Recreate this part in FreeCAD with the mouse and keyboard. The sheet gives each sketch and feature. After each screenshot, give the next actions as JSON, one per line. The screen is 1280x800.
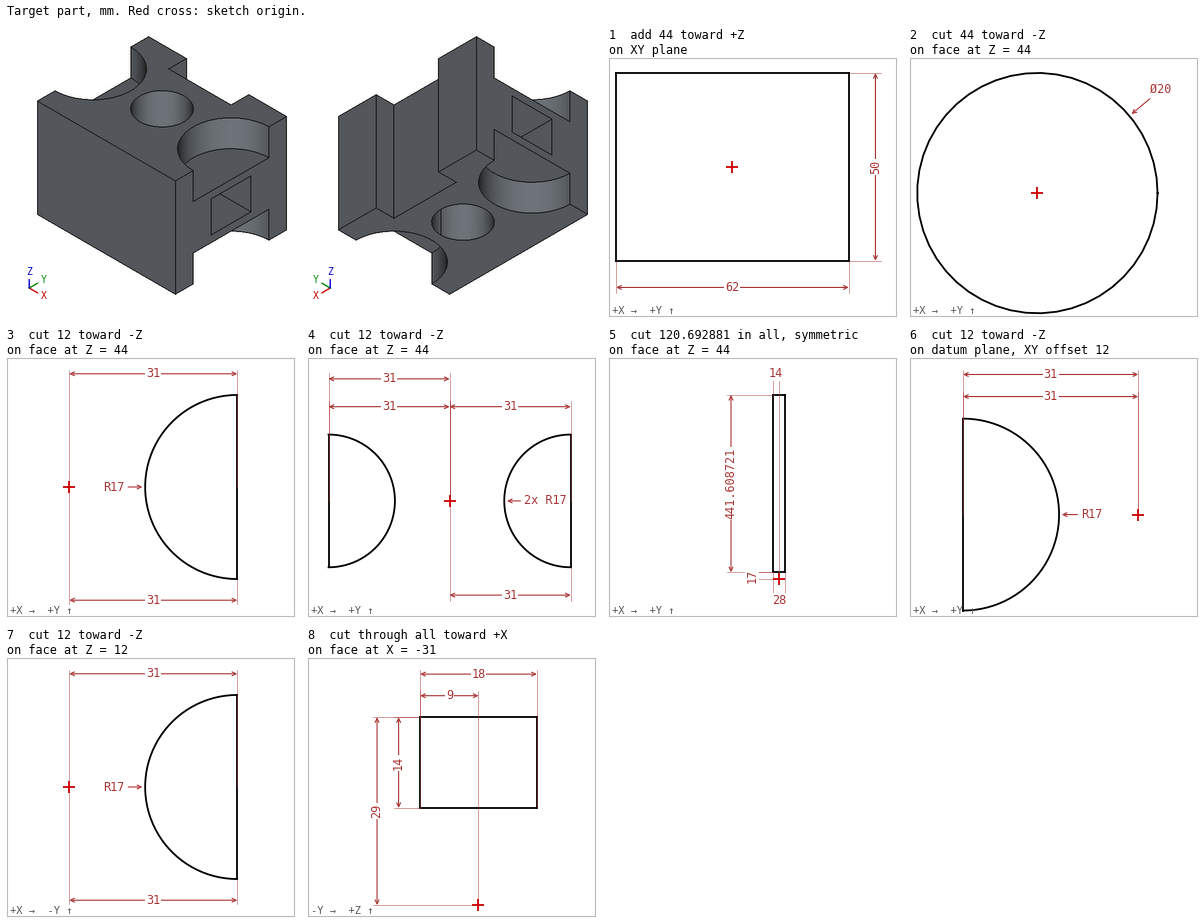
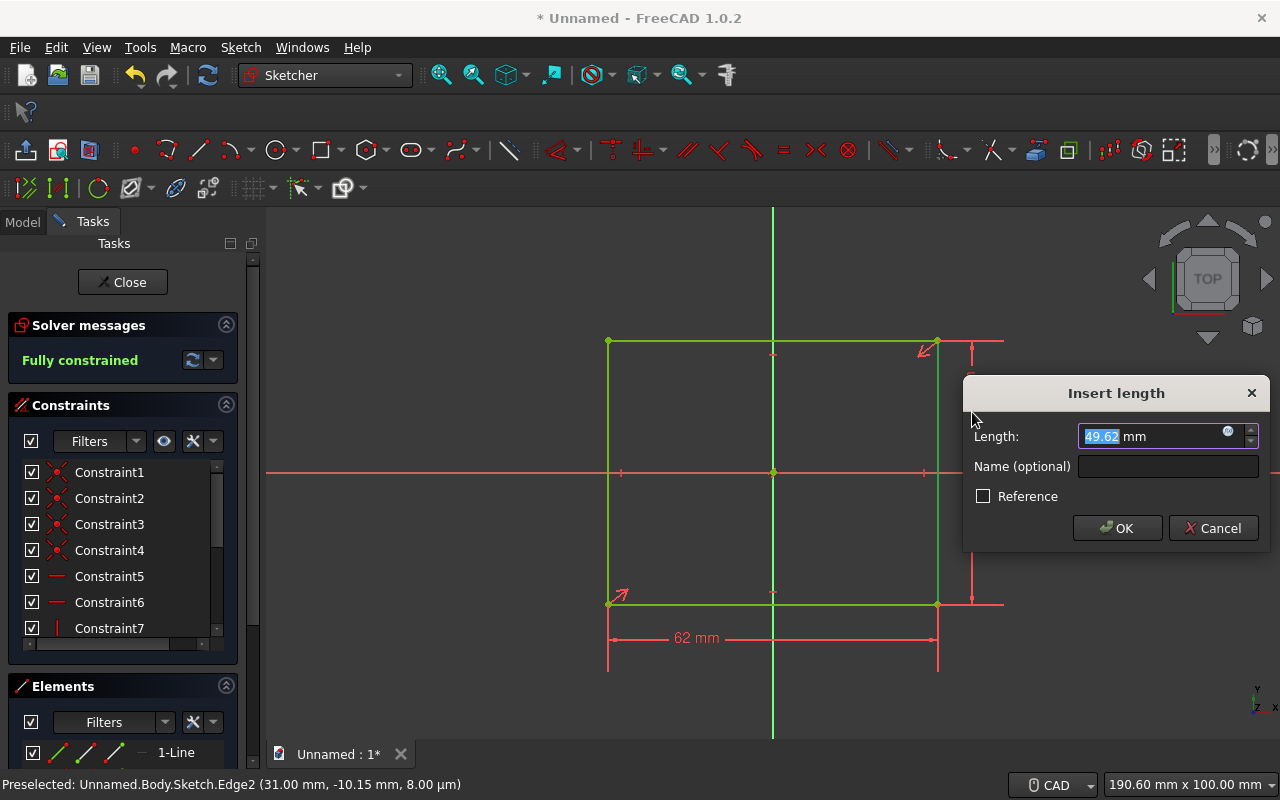
{"action": "type", "text": "50"}
{"action": "key", "text": "Return"}
{"action": "key", "text": "Escape"}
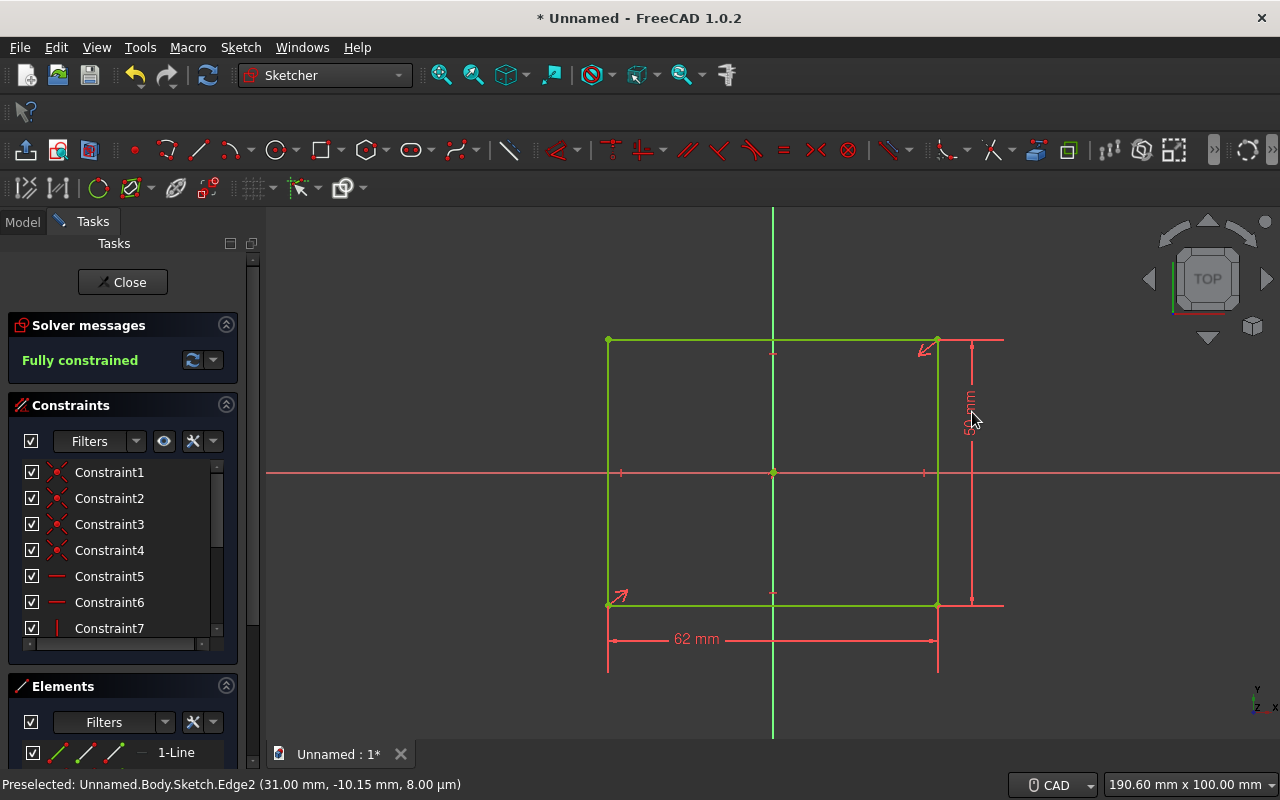
{"action": "left_click", "coordinate": [123, 282]}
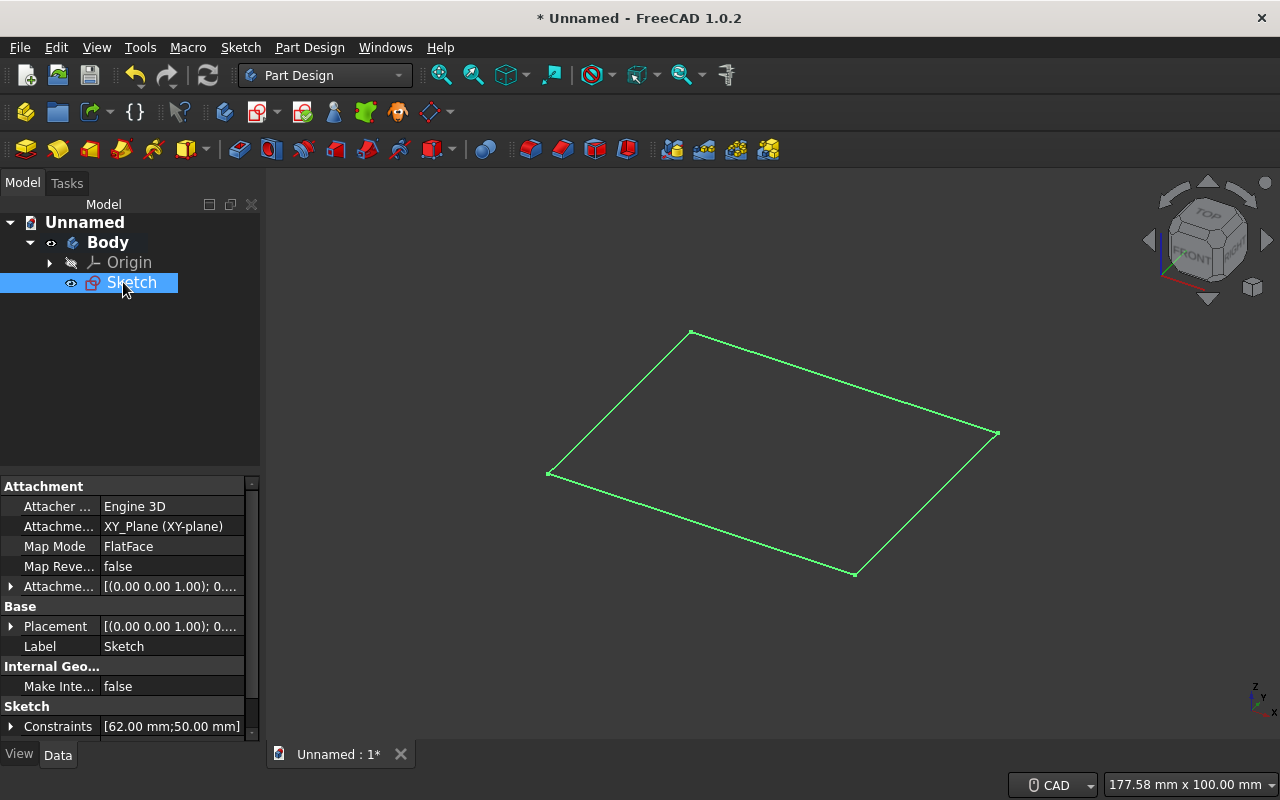
{"action": "left_click", "coordinate": [26, 150]}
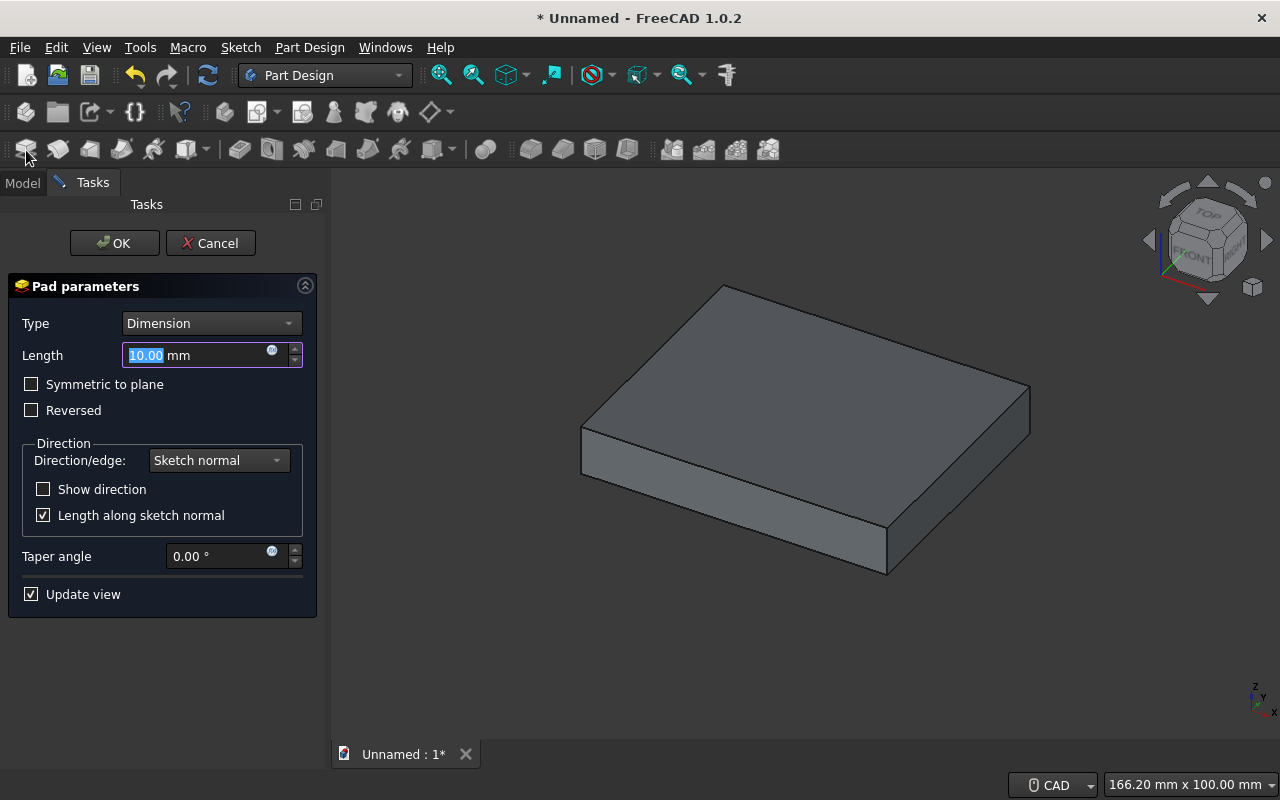
{"action": "type", "text": "44"}
{"action": "key", "text": "Tab"}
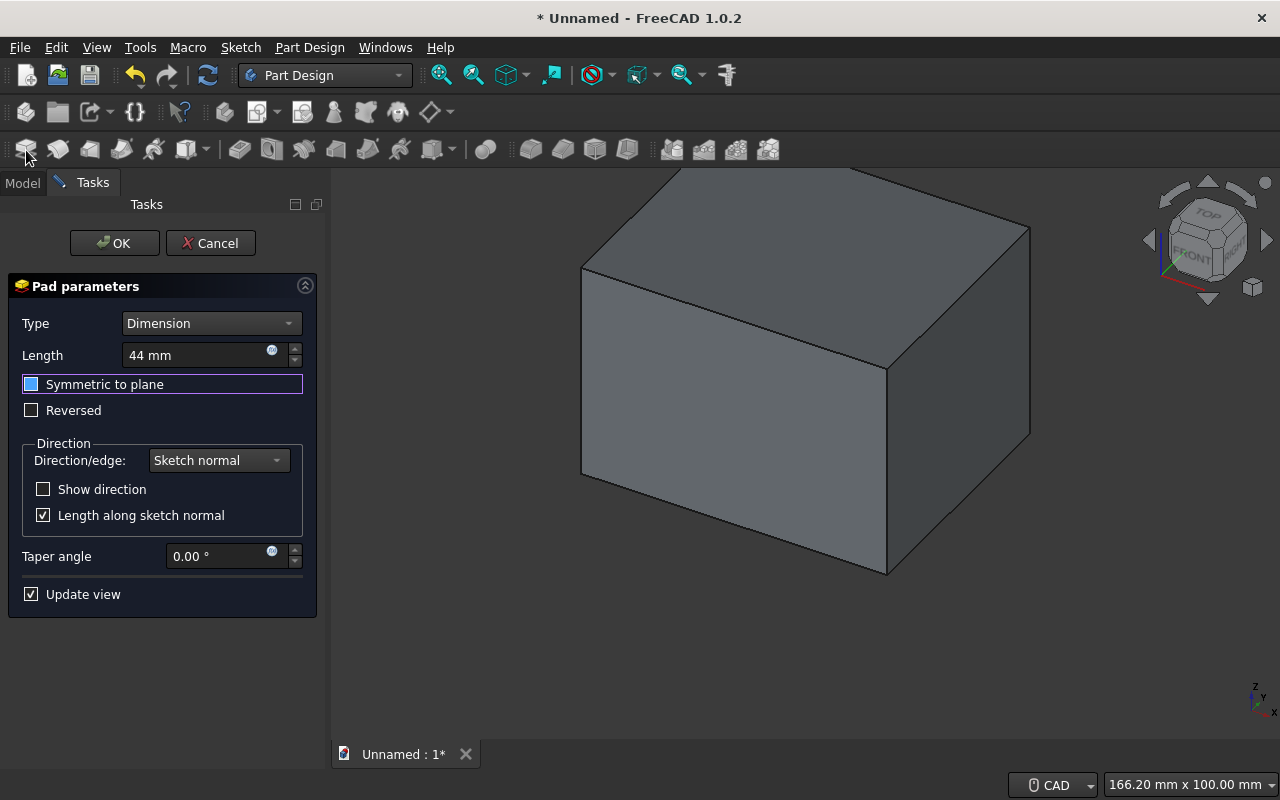
{"action": "left_click", "coordinate": [115, 243]}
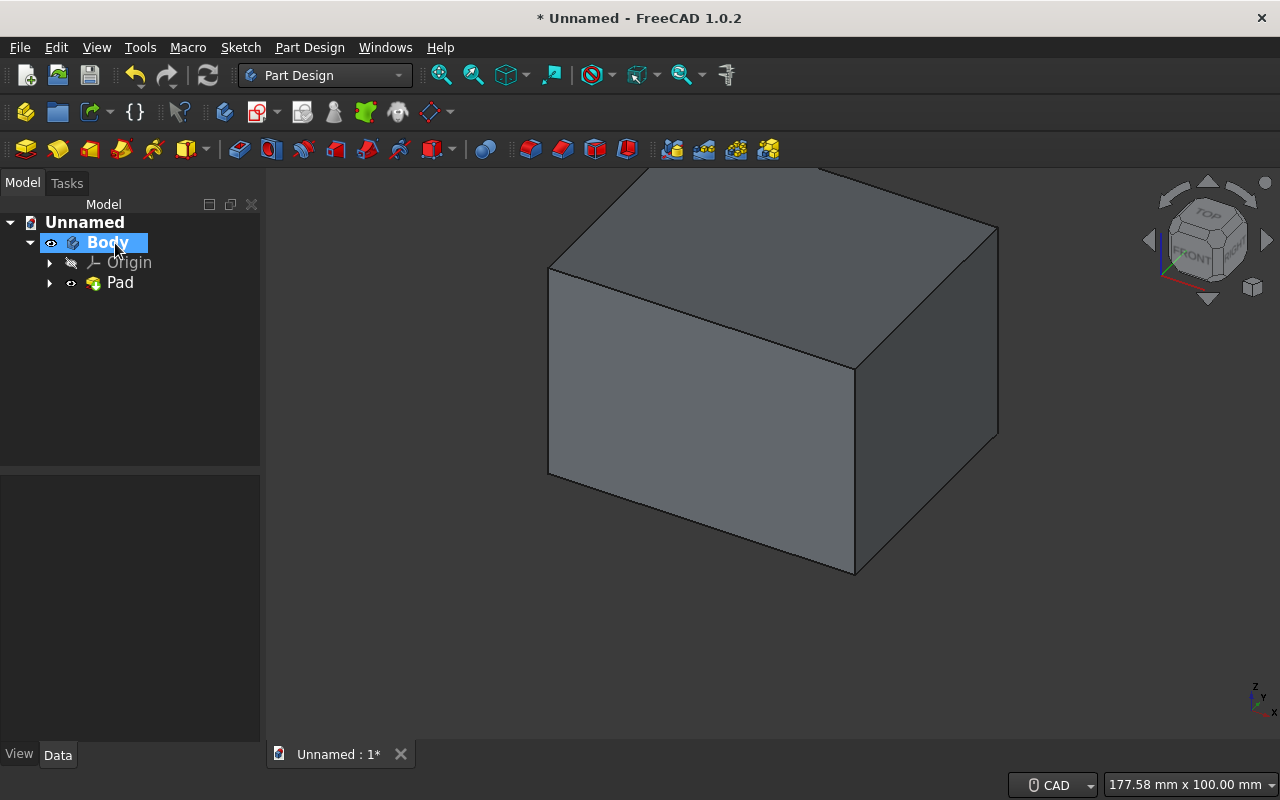
{"action": "key", "text": "v f"}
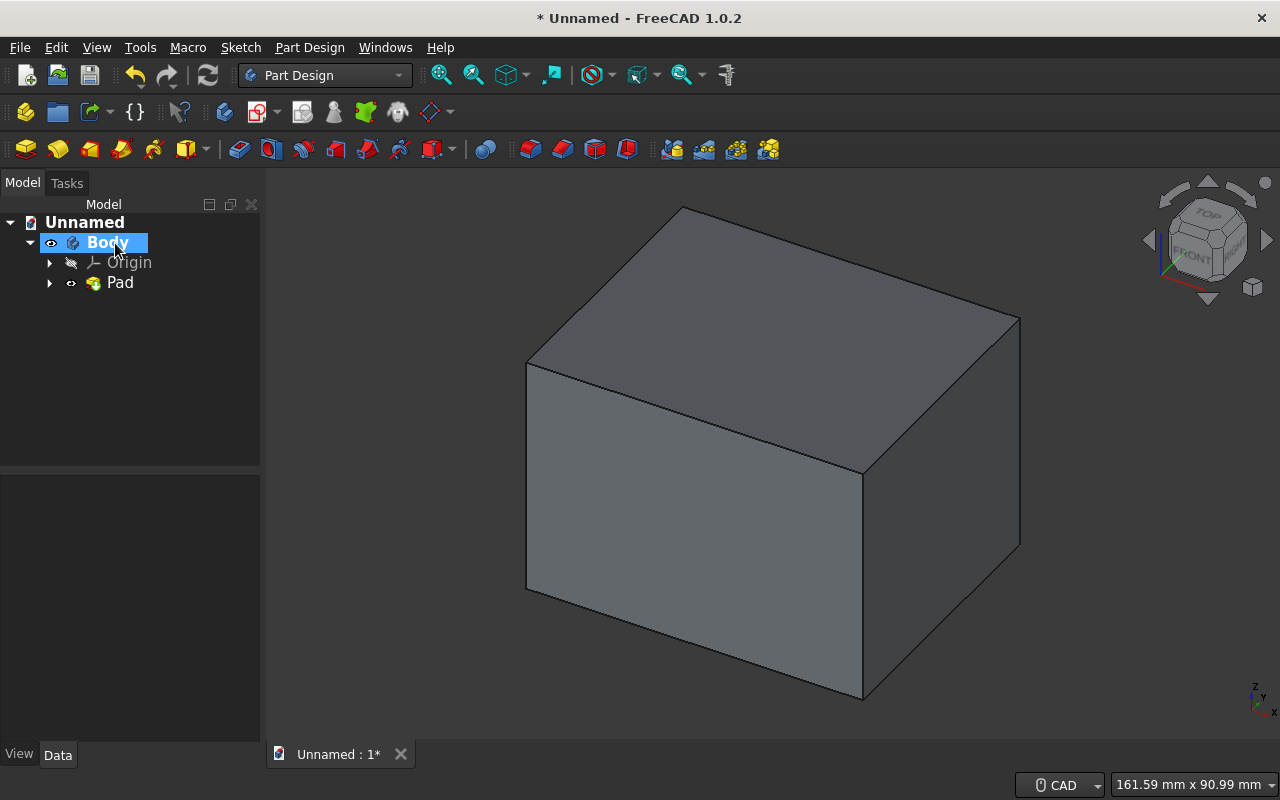
{"action": "left_click", "coordinate": [773, 339]}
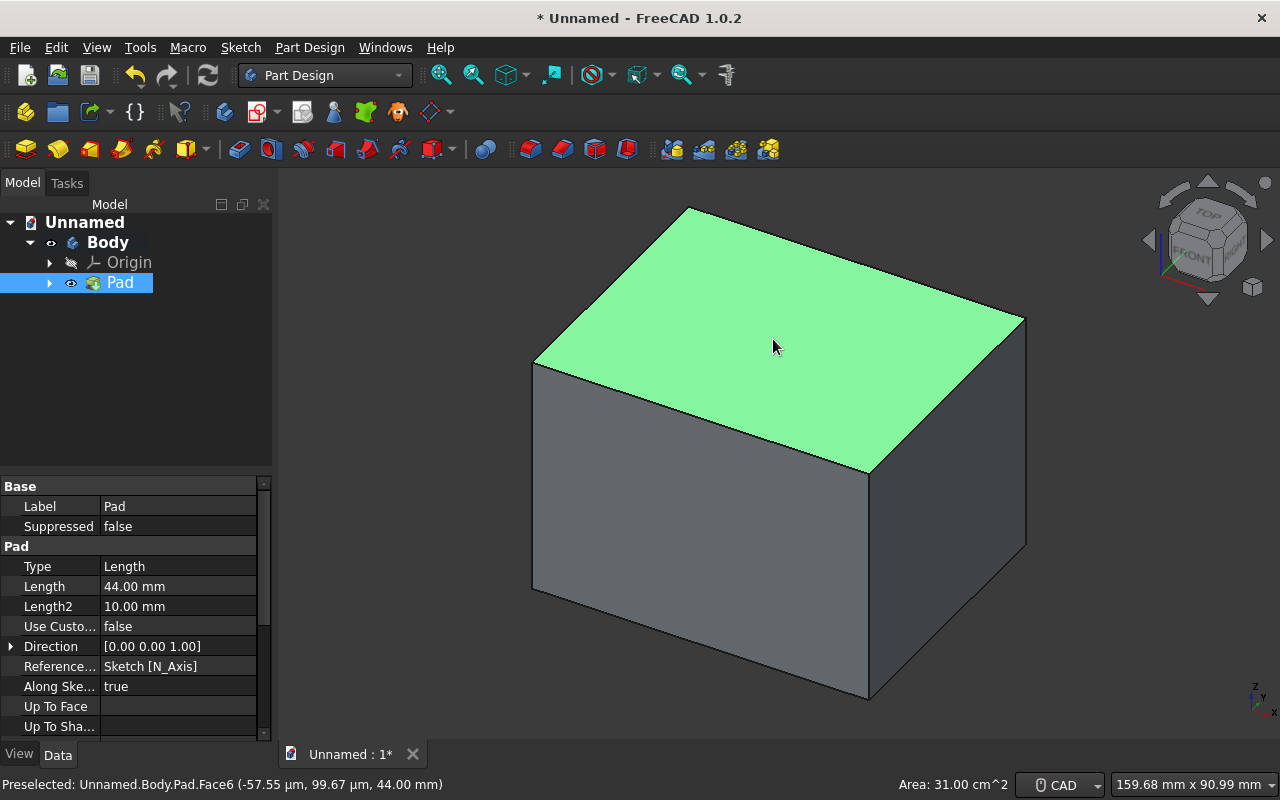
{"action": "left_click", "coordinate": [258, 112]}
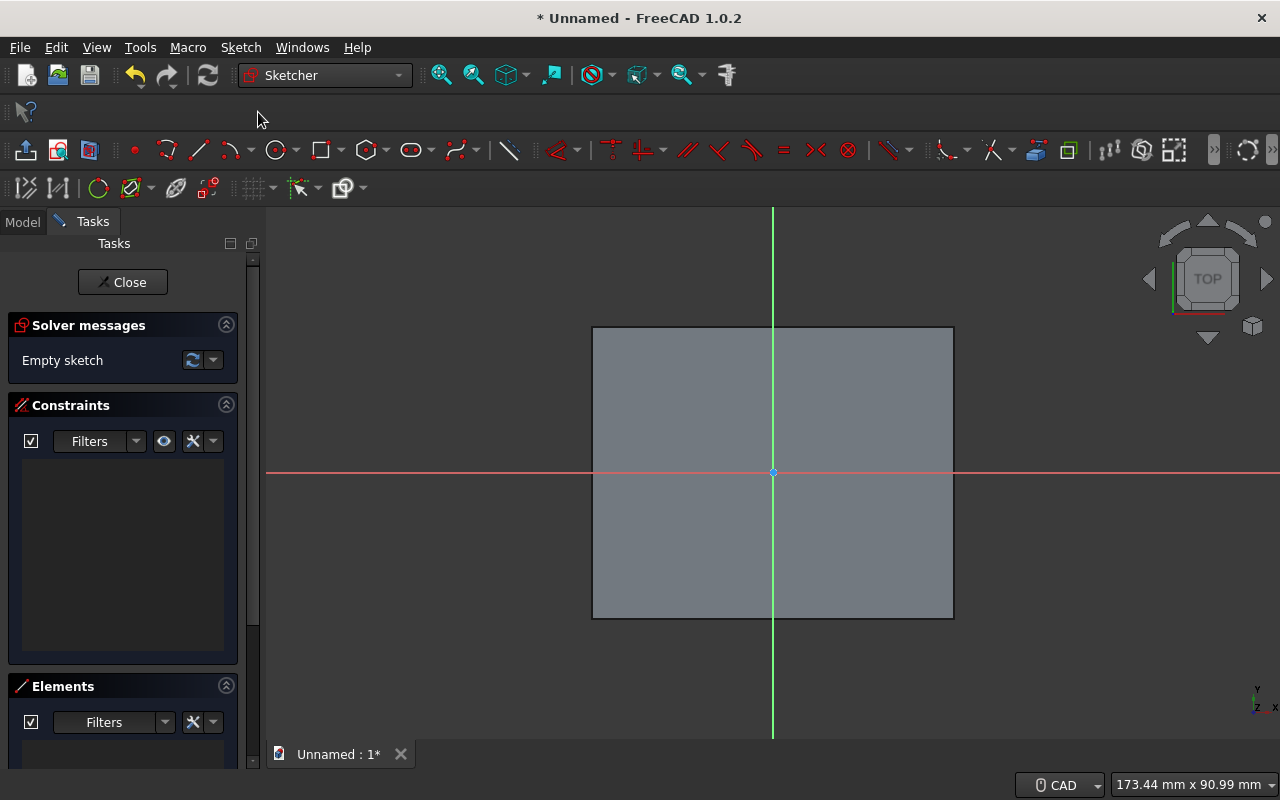
{"action": "scroll", "coordinate": [813, 473], "scroll_direction": "up", "scroll_amount": 5}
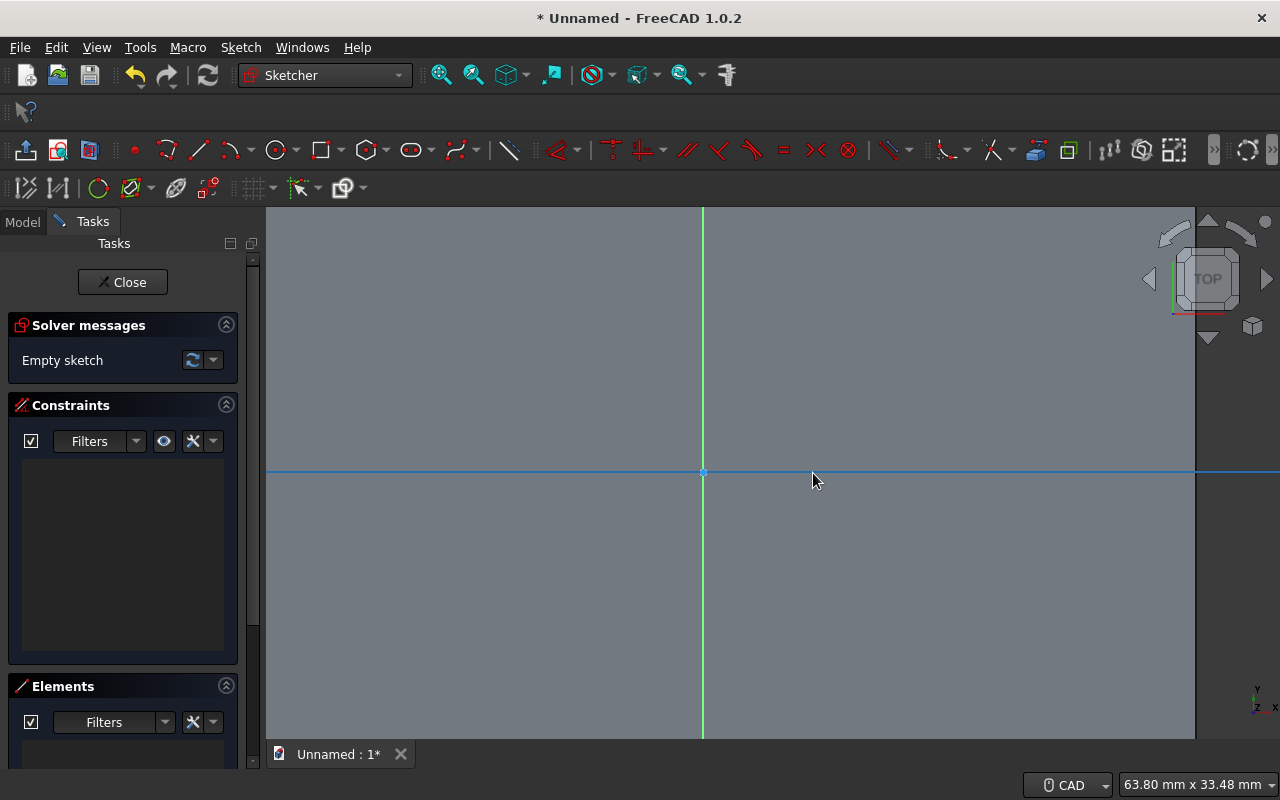
{"action": "key", "text": "g c"}